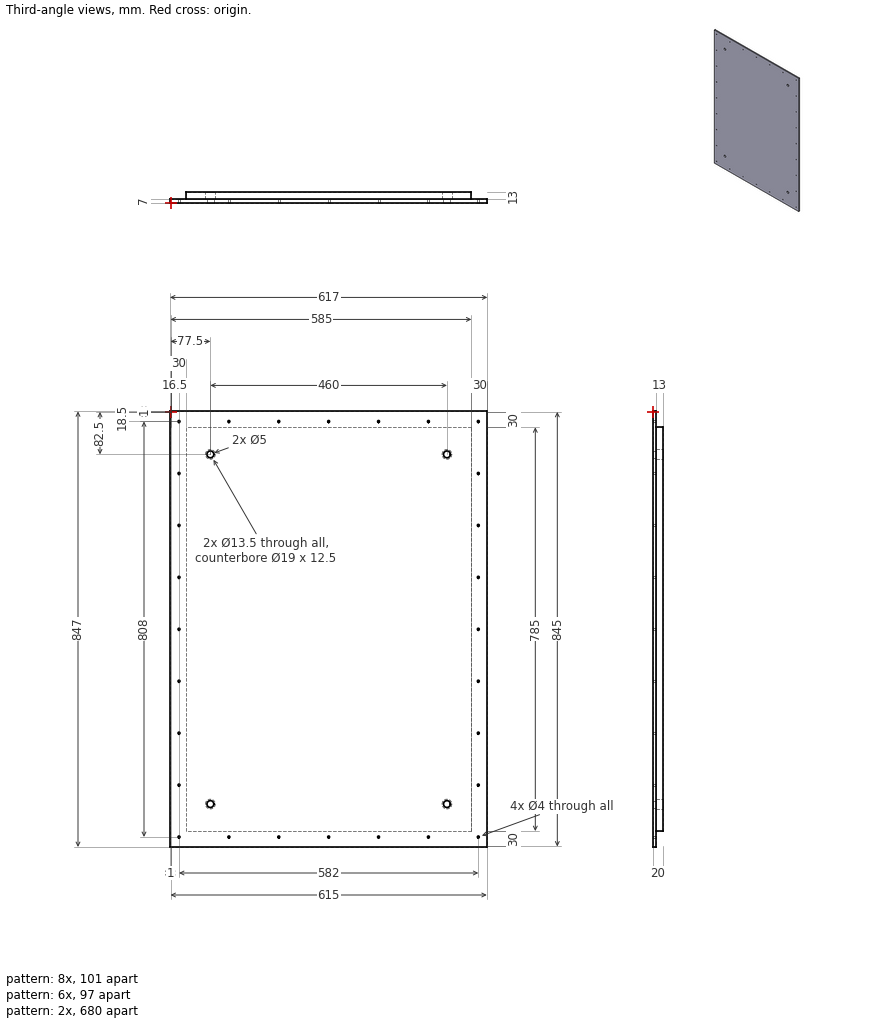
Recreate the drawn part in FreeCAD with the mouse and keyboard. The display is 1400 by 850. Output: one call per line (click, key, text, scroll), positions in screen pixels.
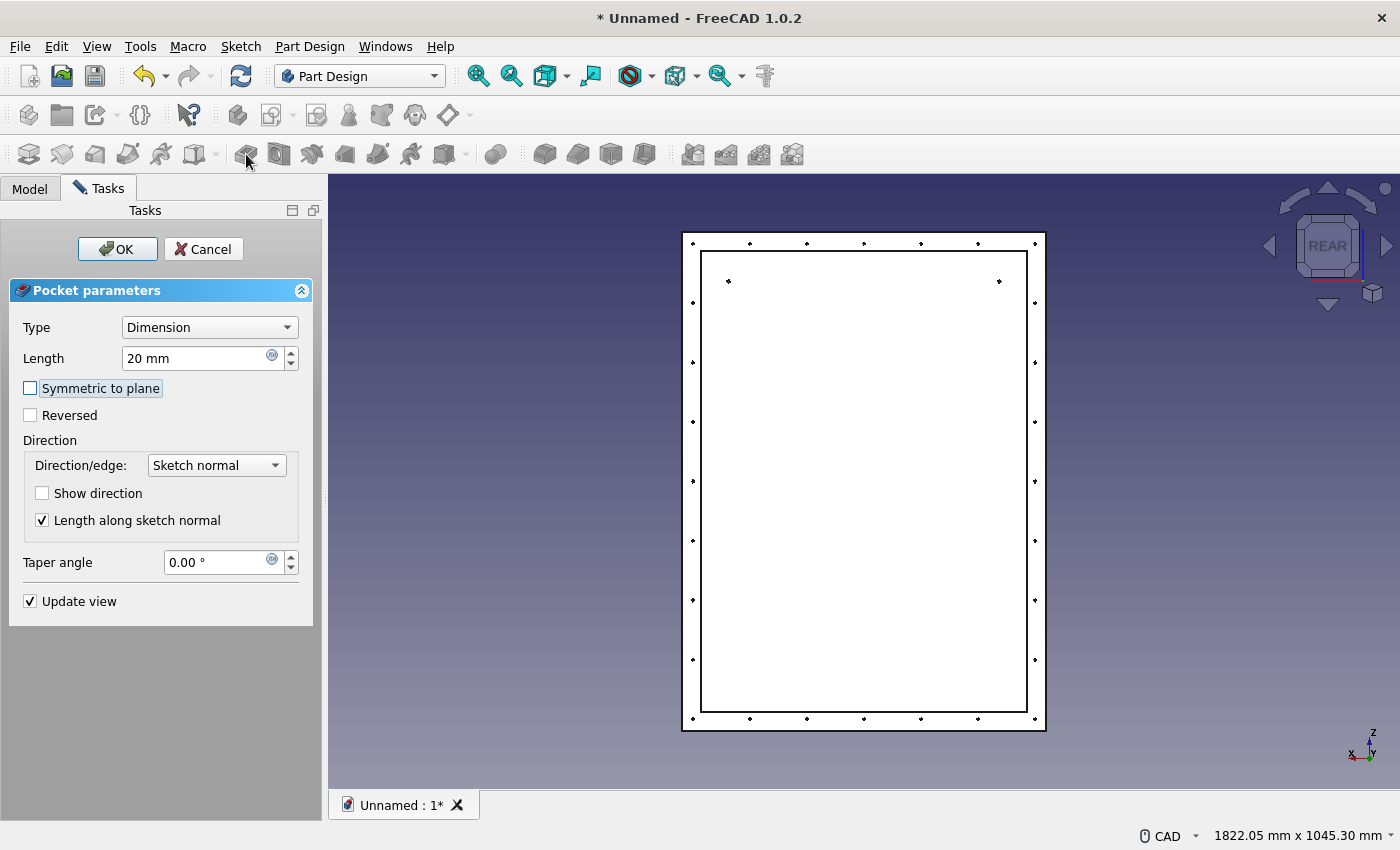
click(118, 249)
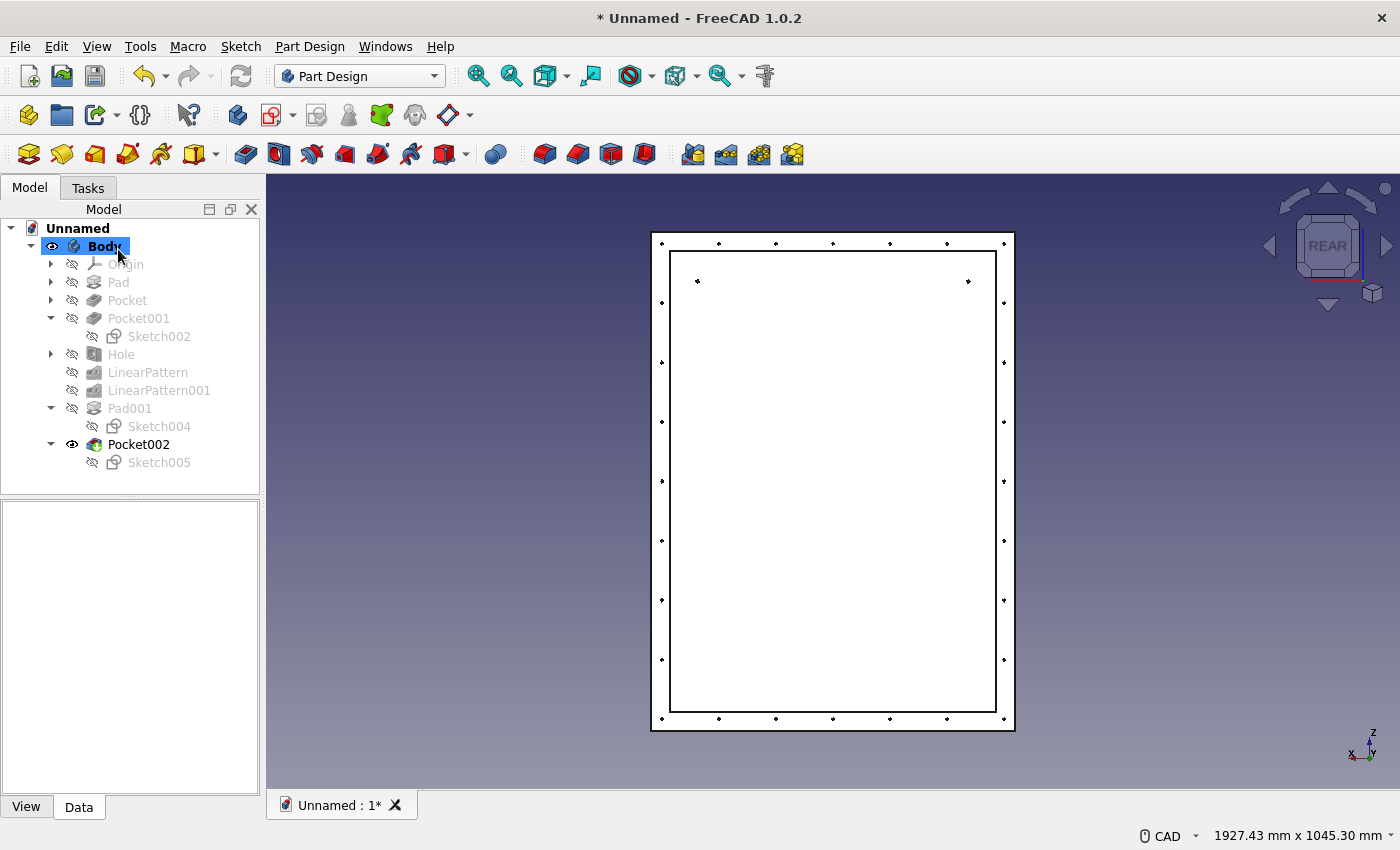
click(833, 415)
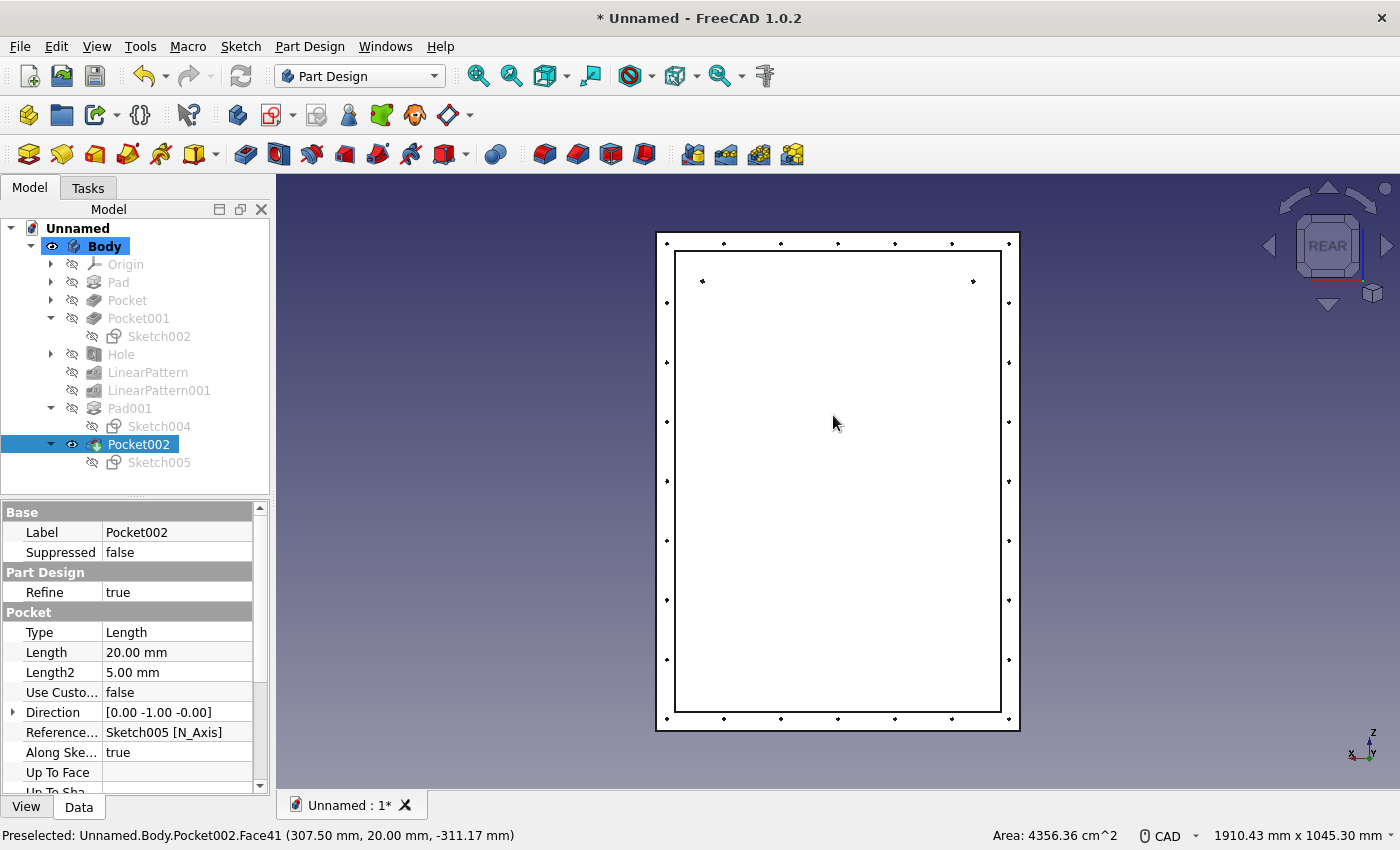
click(270, 116)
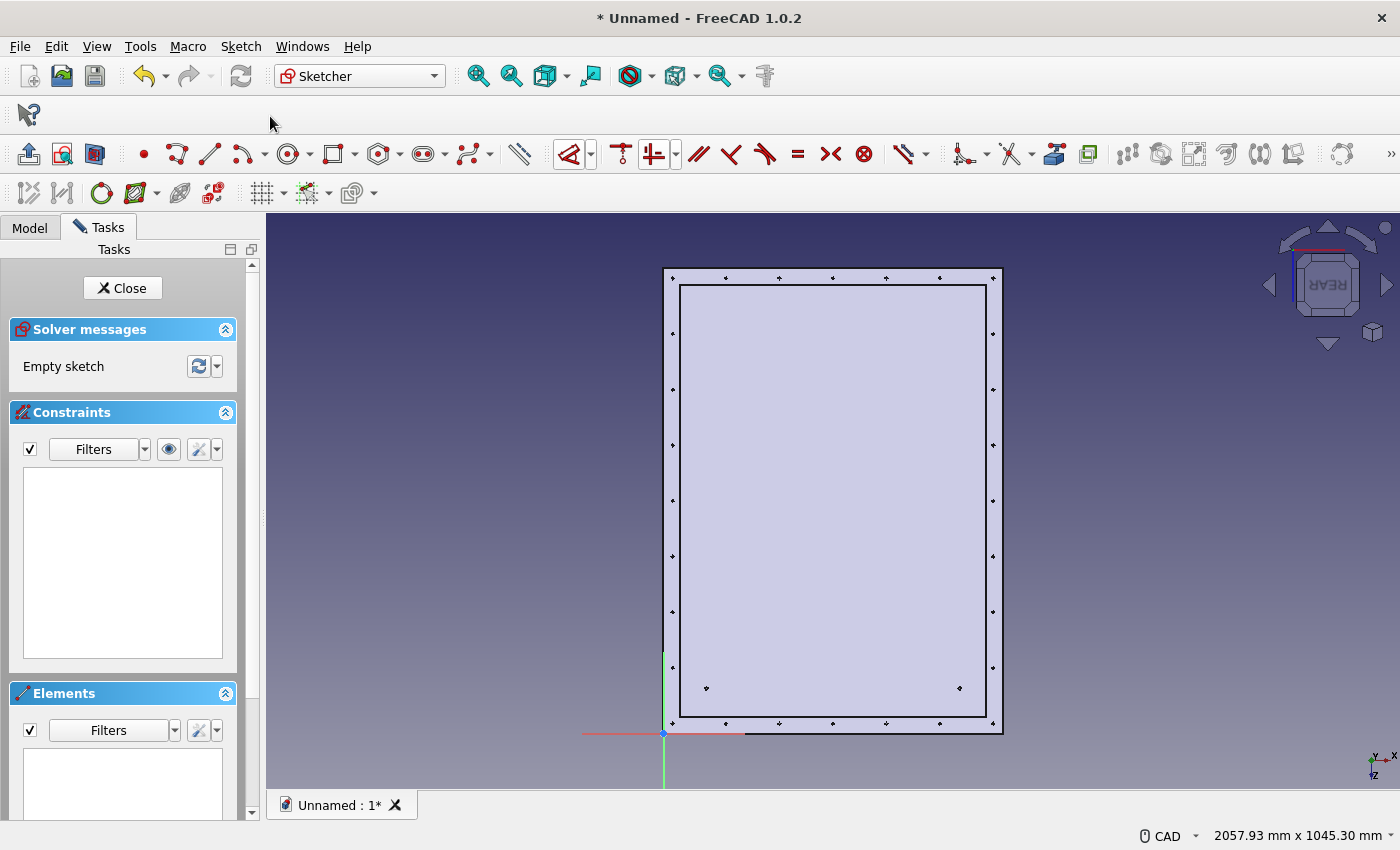
scroll(853, 761, up, 4)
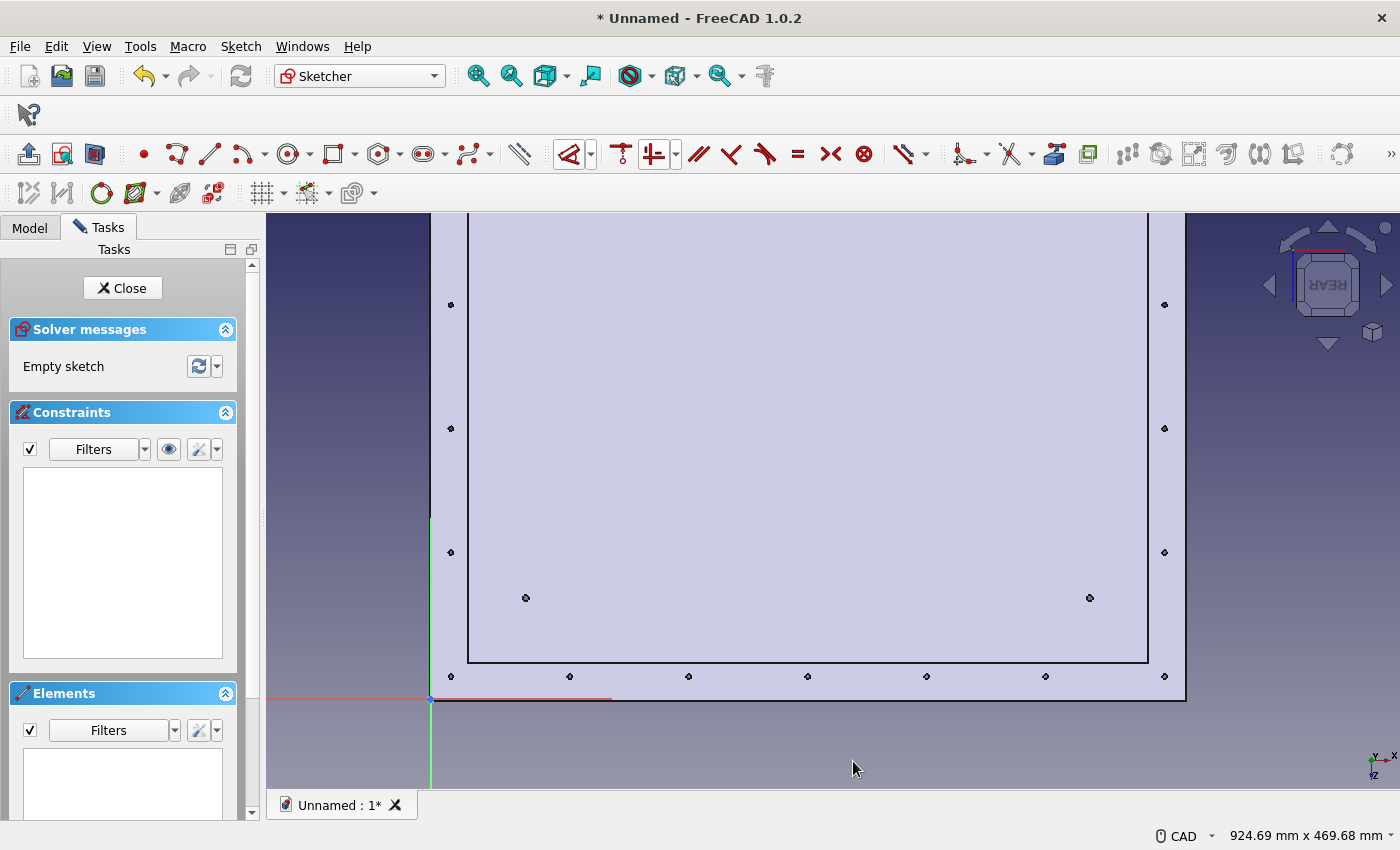
click(288, 154)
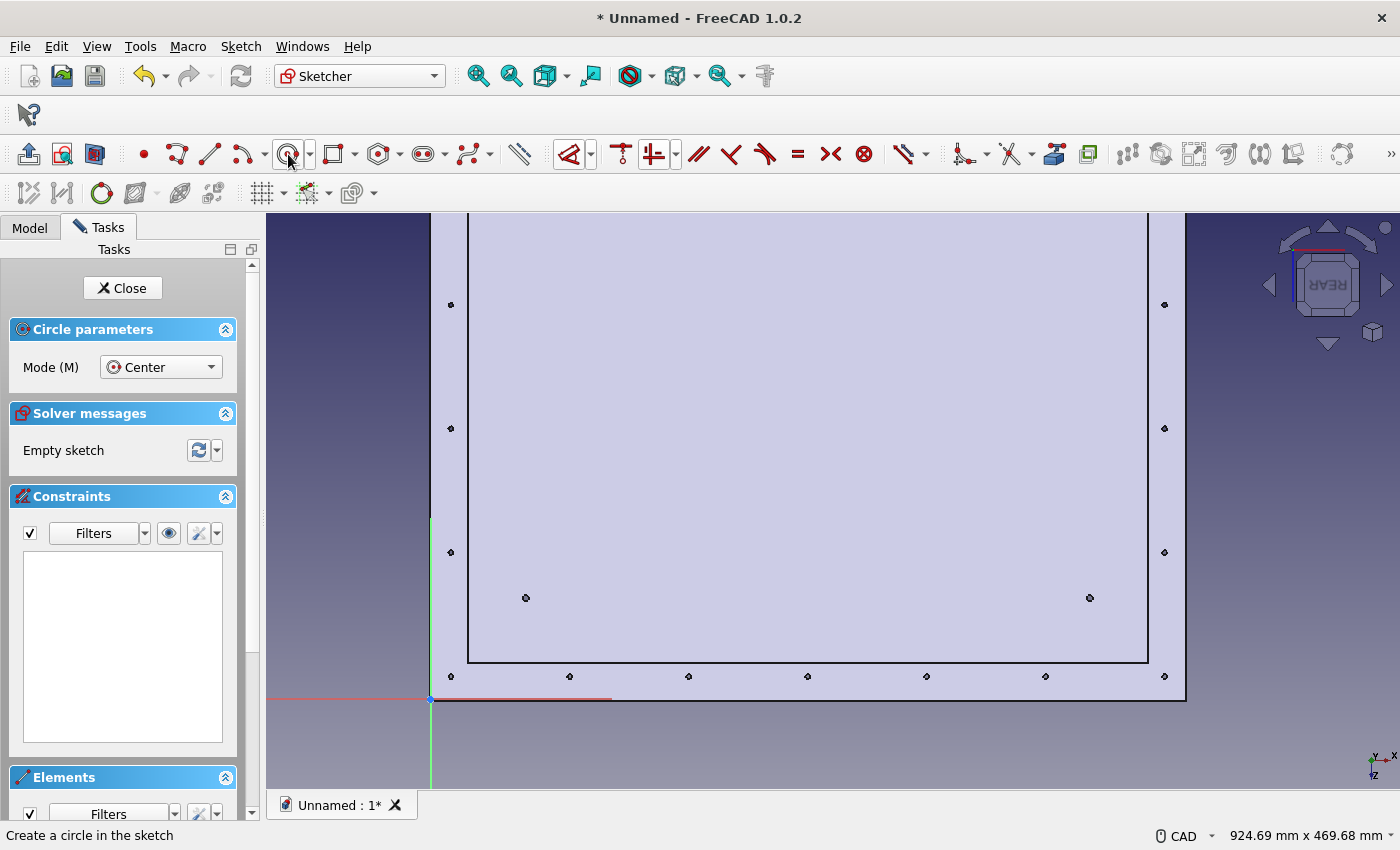
scroll(526, 598, up, 6)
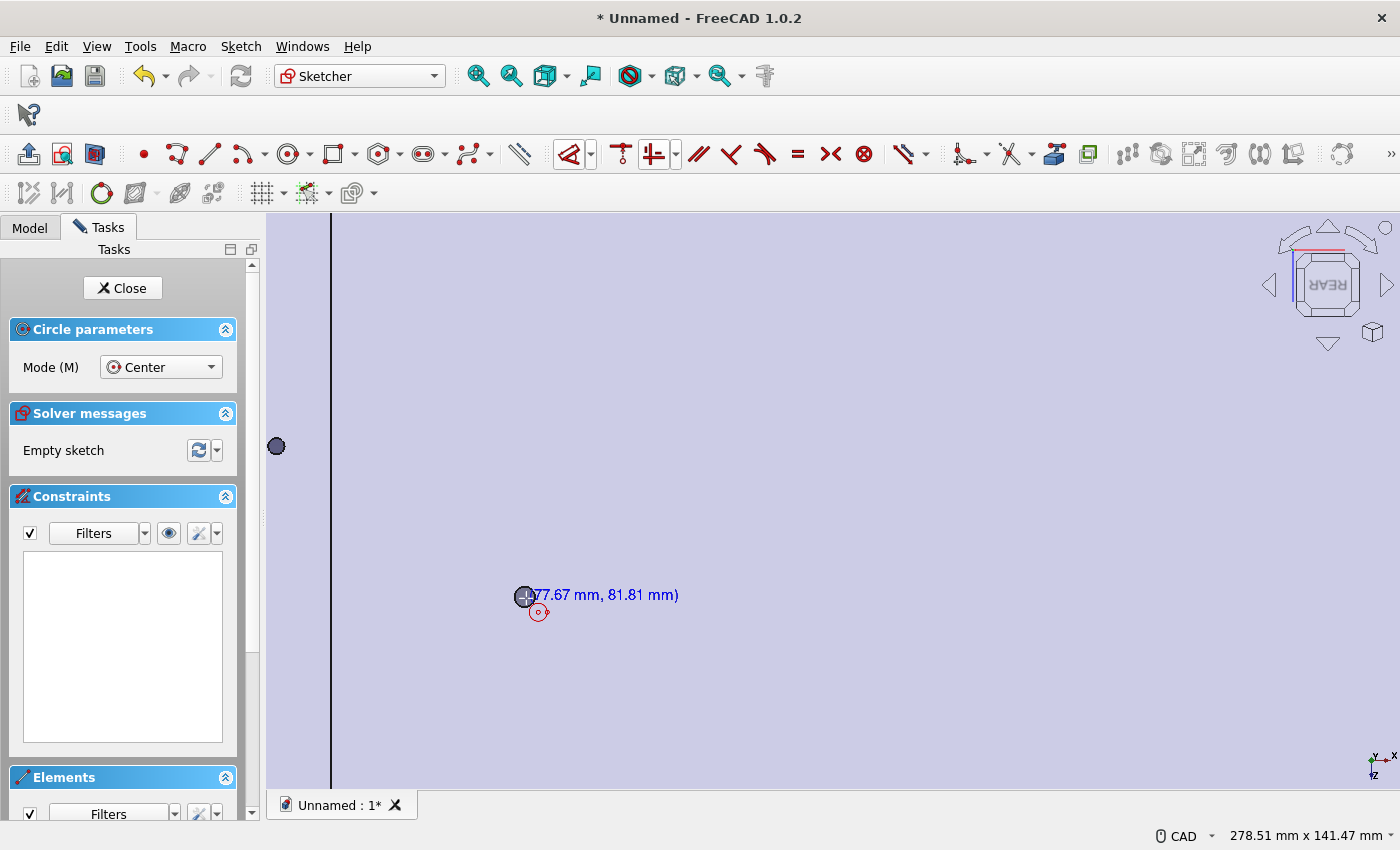
click(525, 597)
move(544, 578)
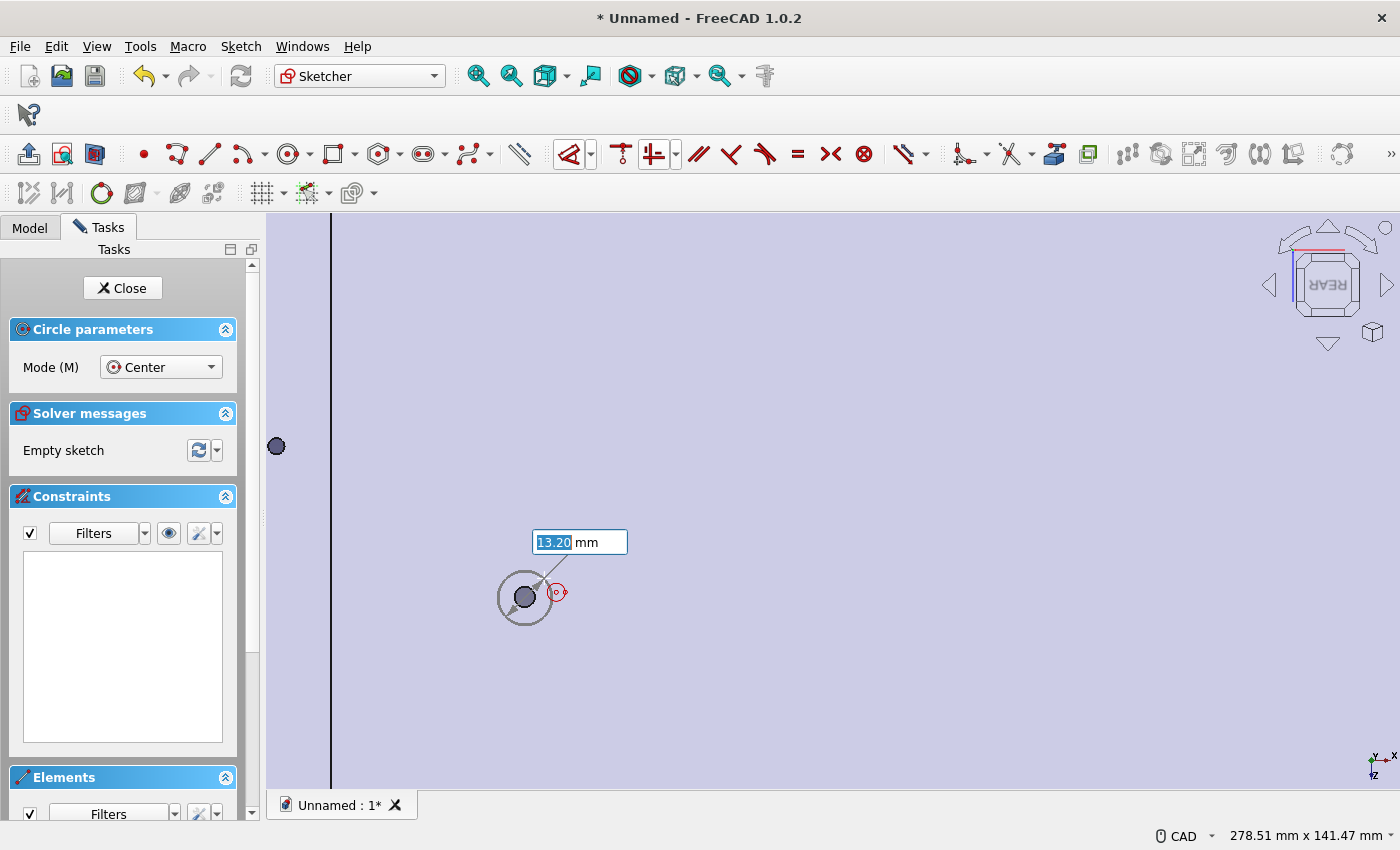
text(13.5)
key(Return)